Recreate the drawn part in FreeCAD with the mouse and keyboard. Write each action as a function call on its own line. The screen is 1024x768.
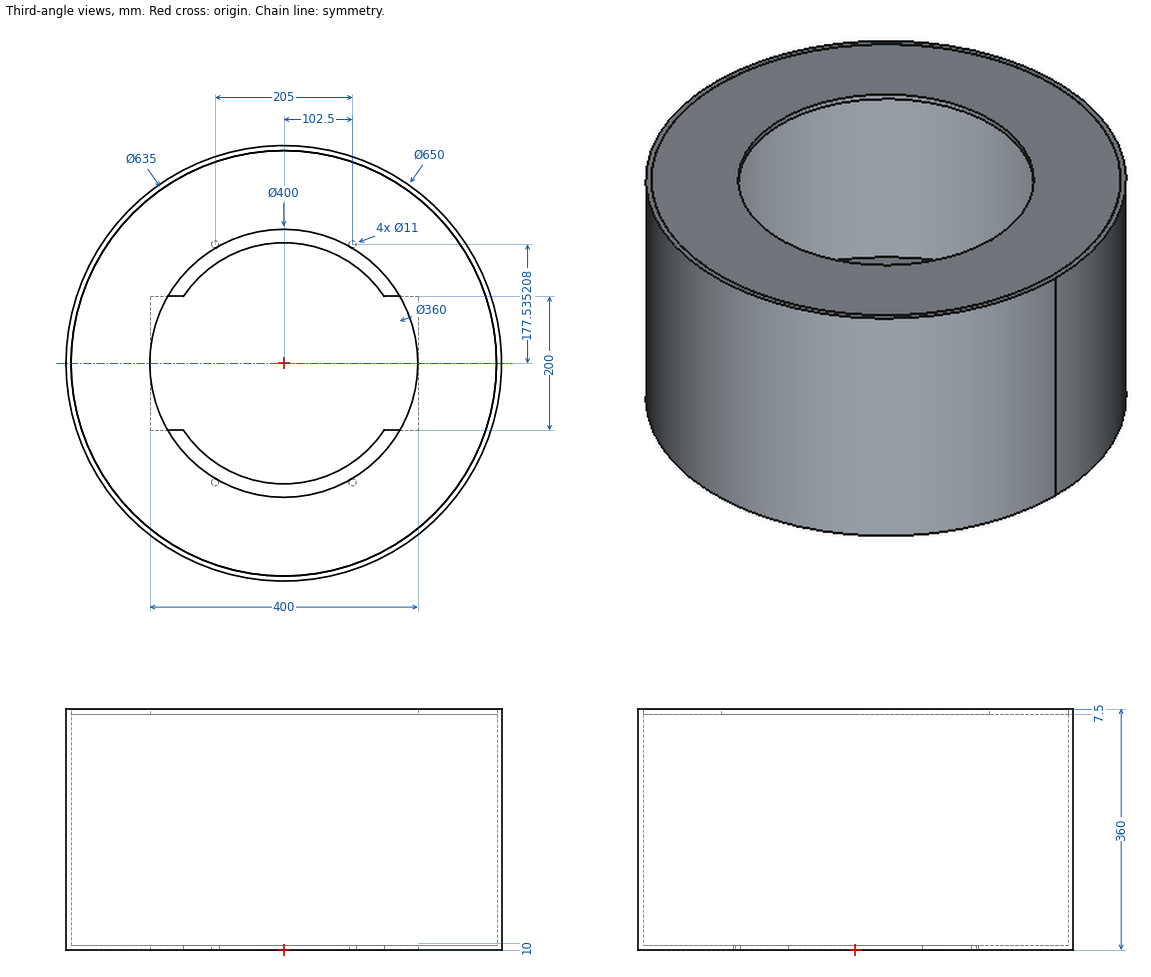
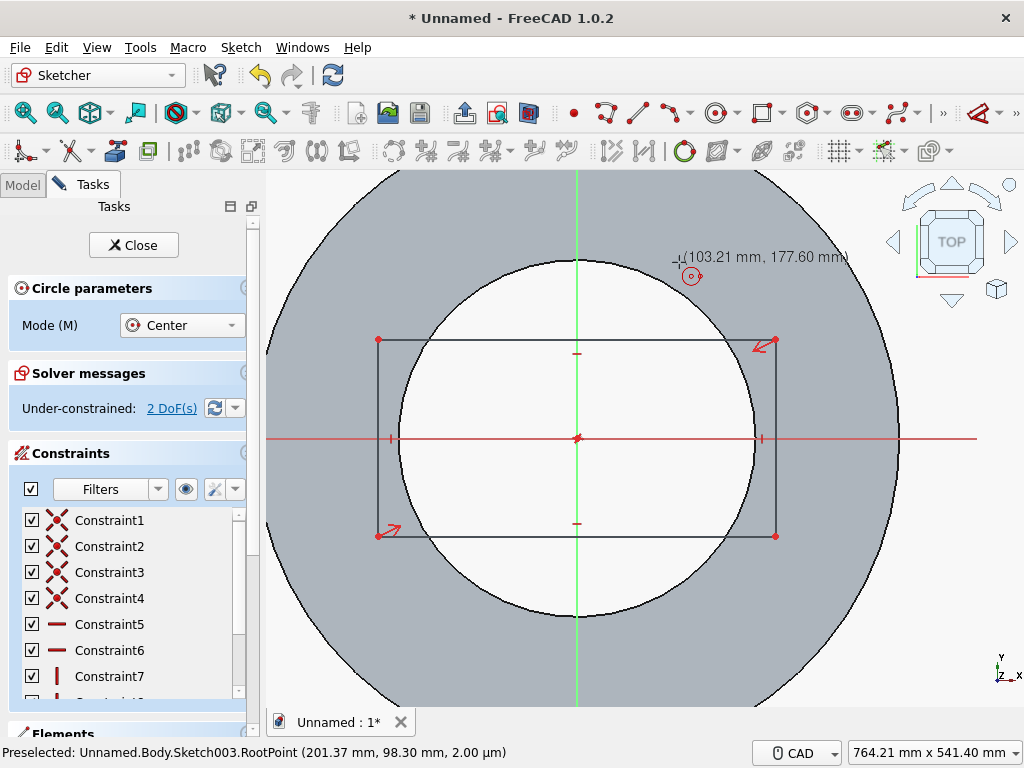
click(679, 262)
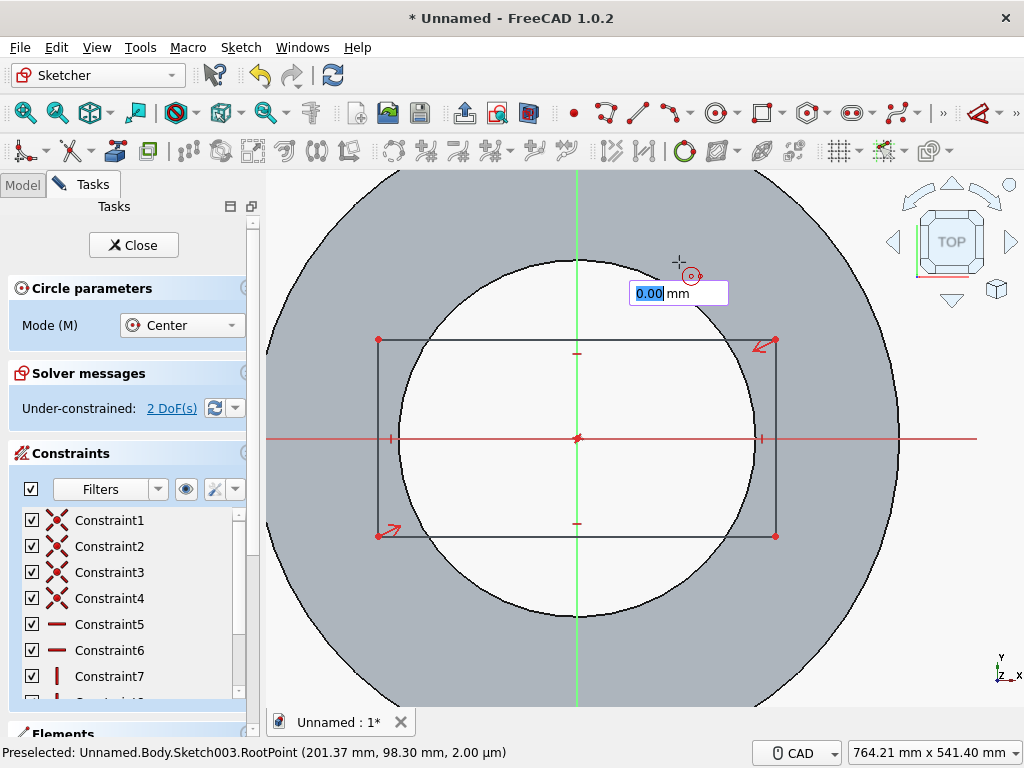
scroll(683, 259, up, 6)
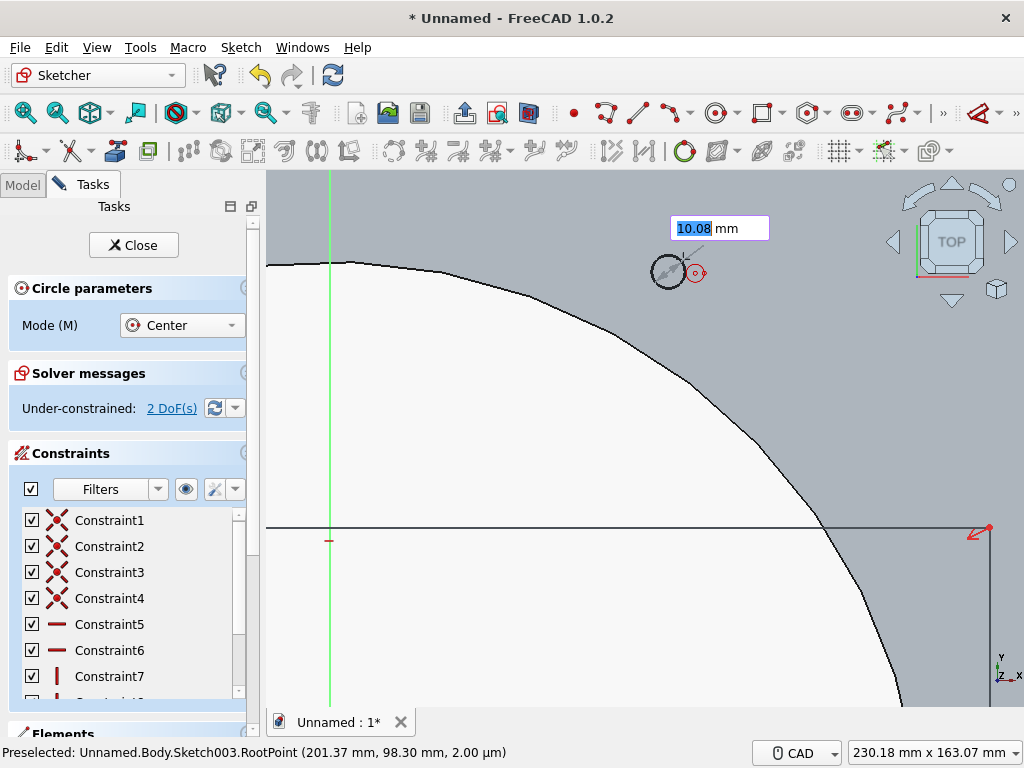
click(680, 257)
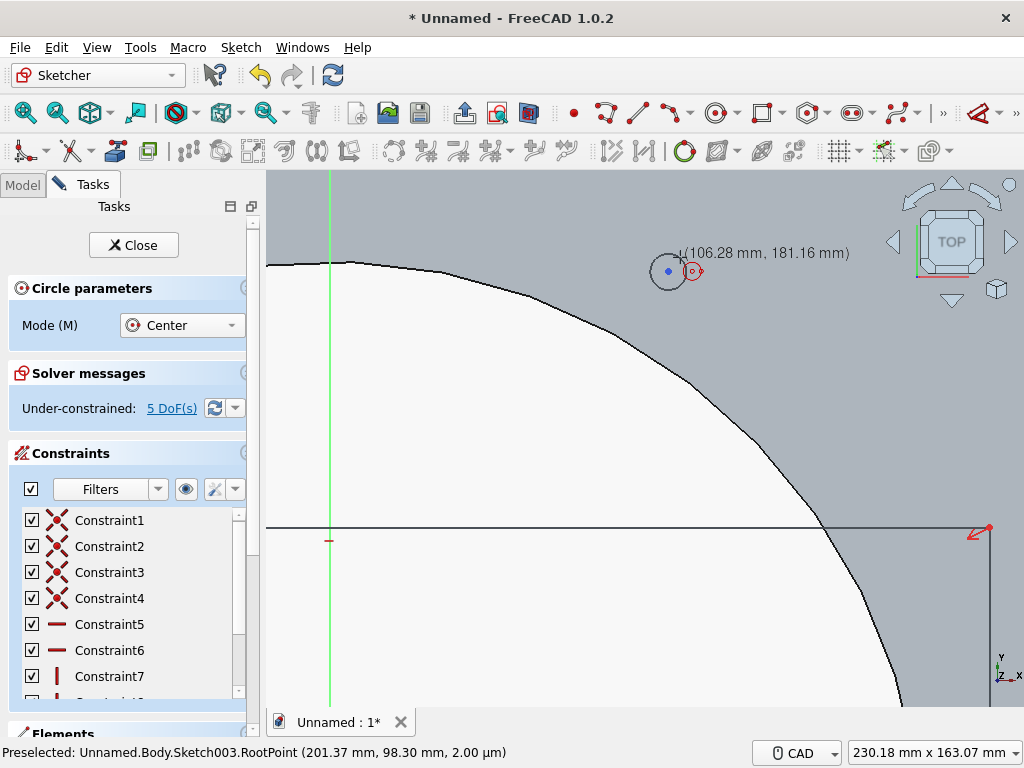
scroll(683, 259, down, 6)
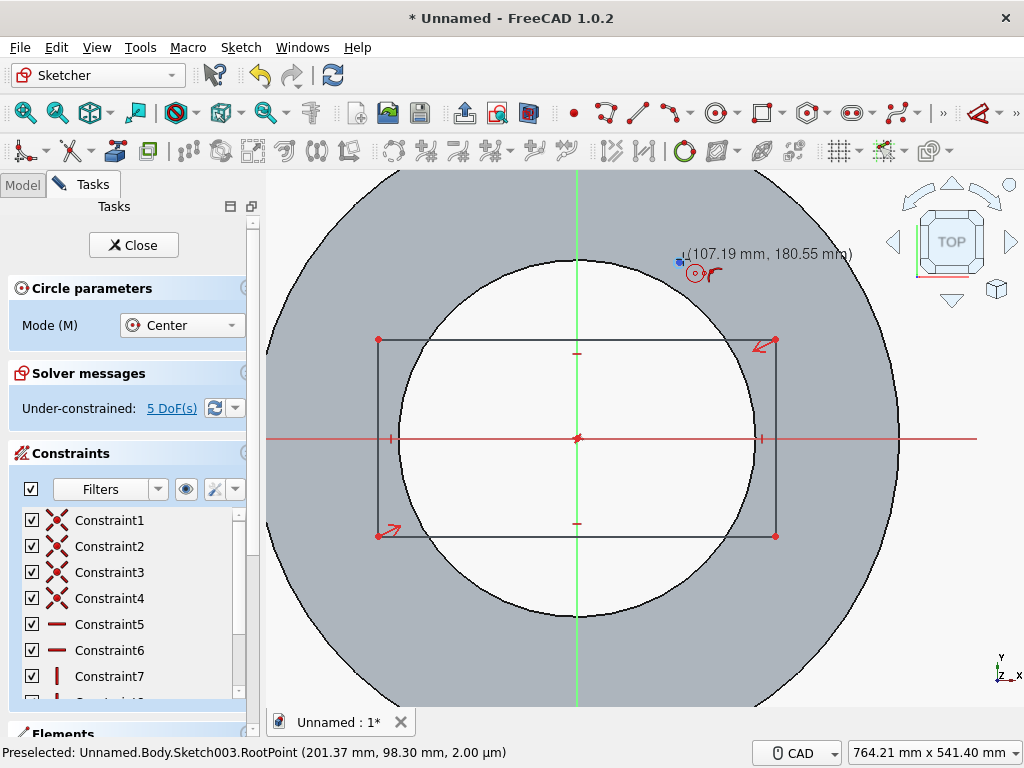
scroll(475, 262, up, 8)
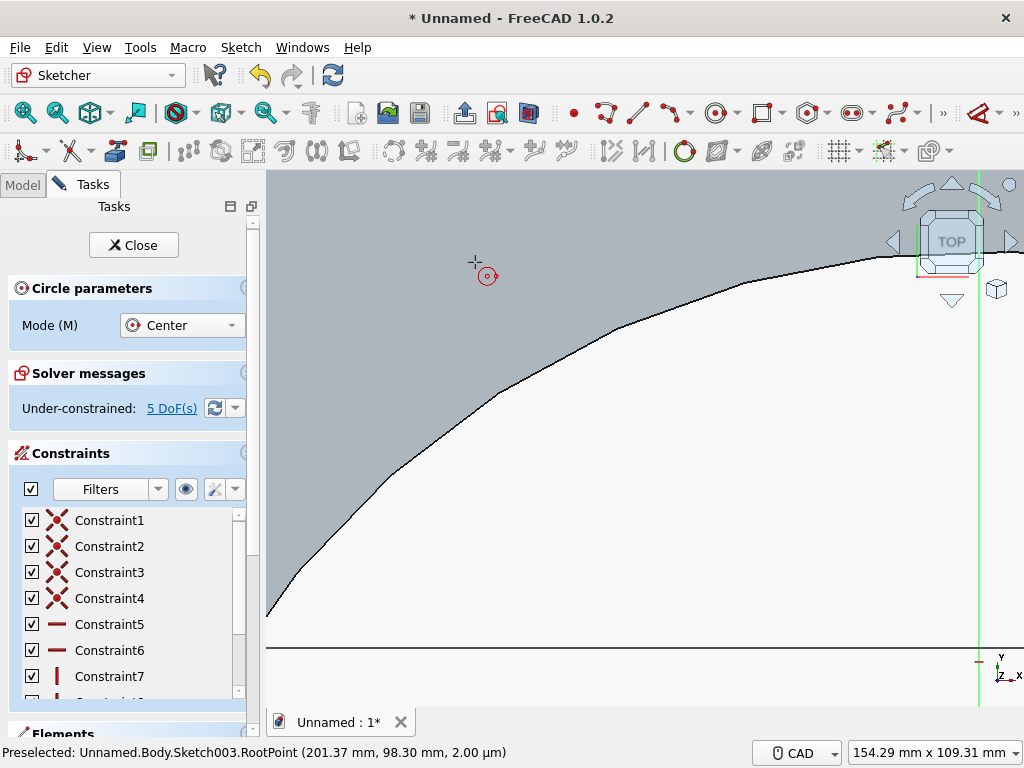
scroll(475, 262, down, 8)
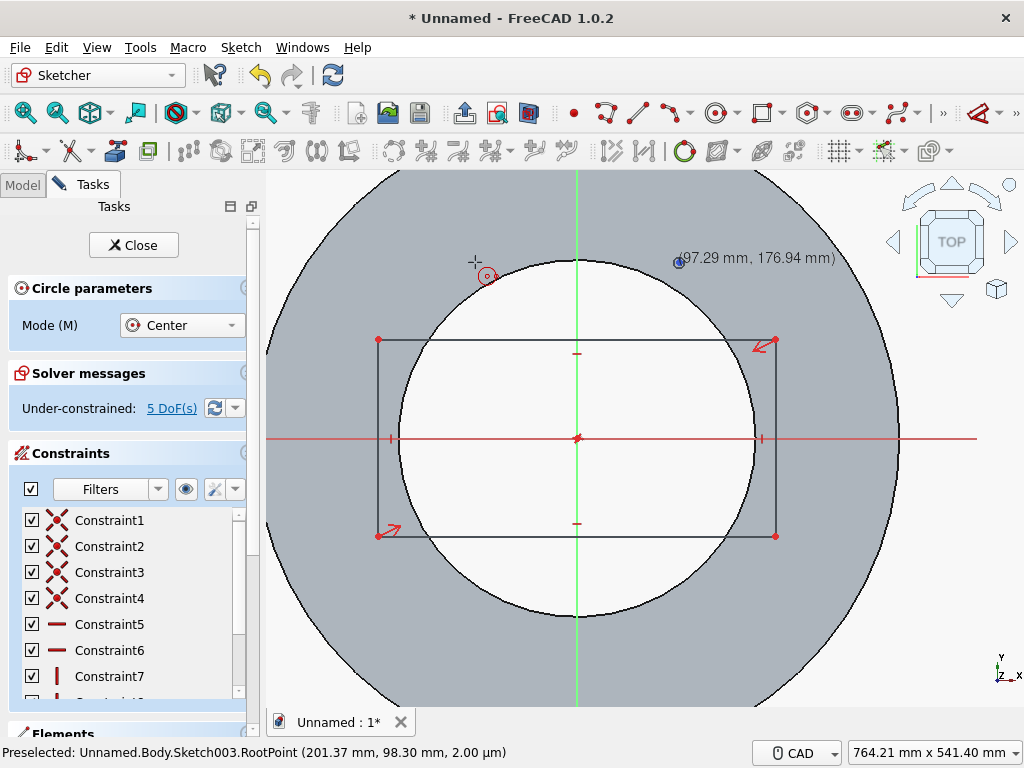
click(475, 262)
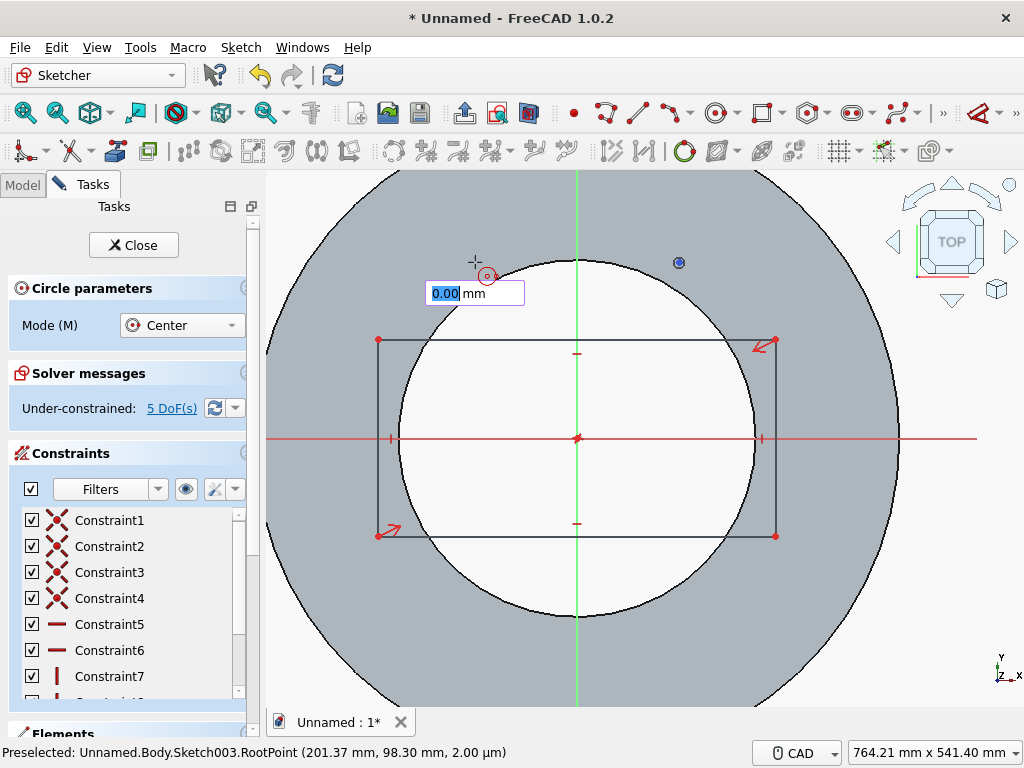
scroll(479, 259, up, 6)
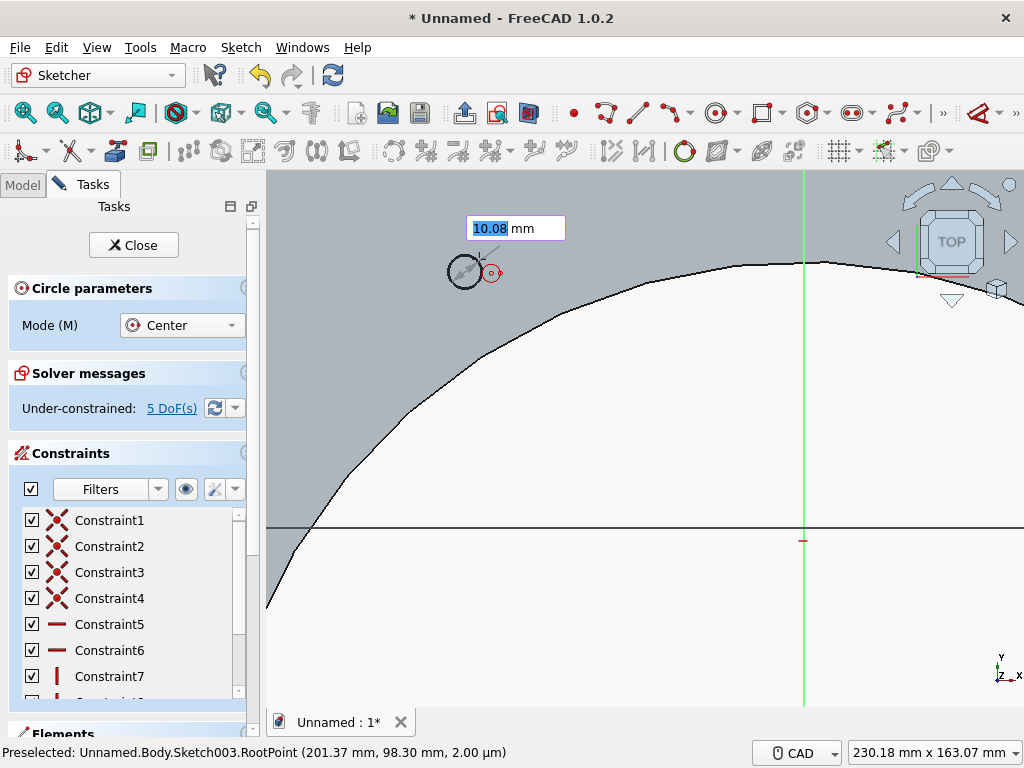
click(479, 257)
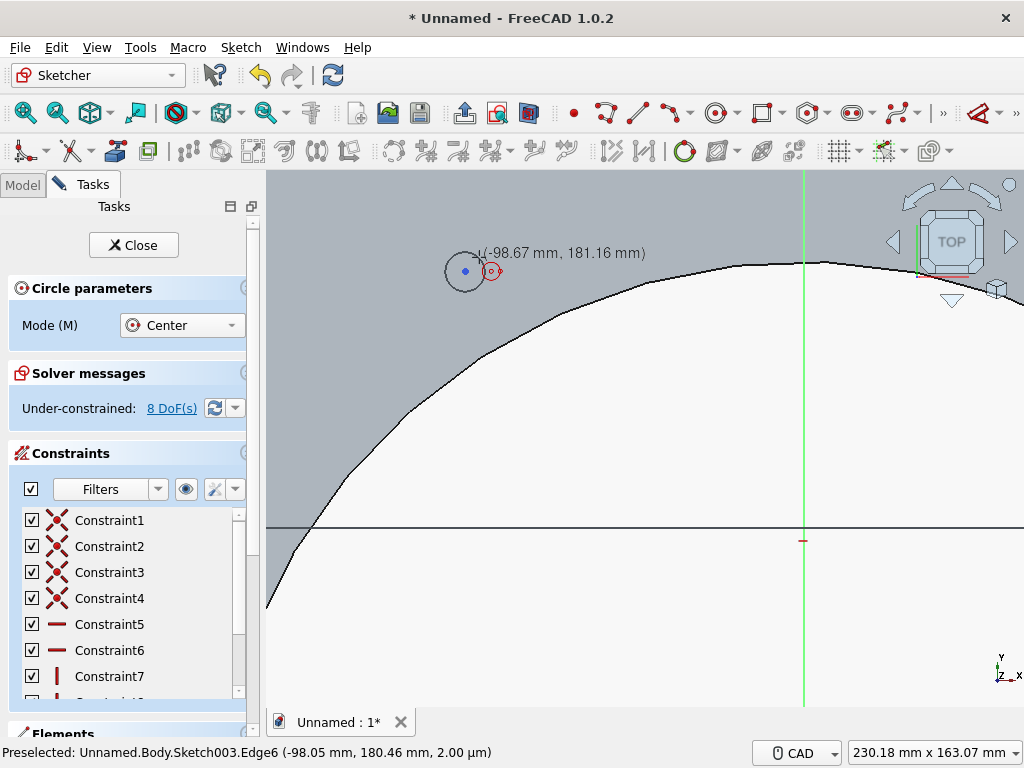
scroll(478, 259, down, 6)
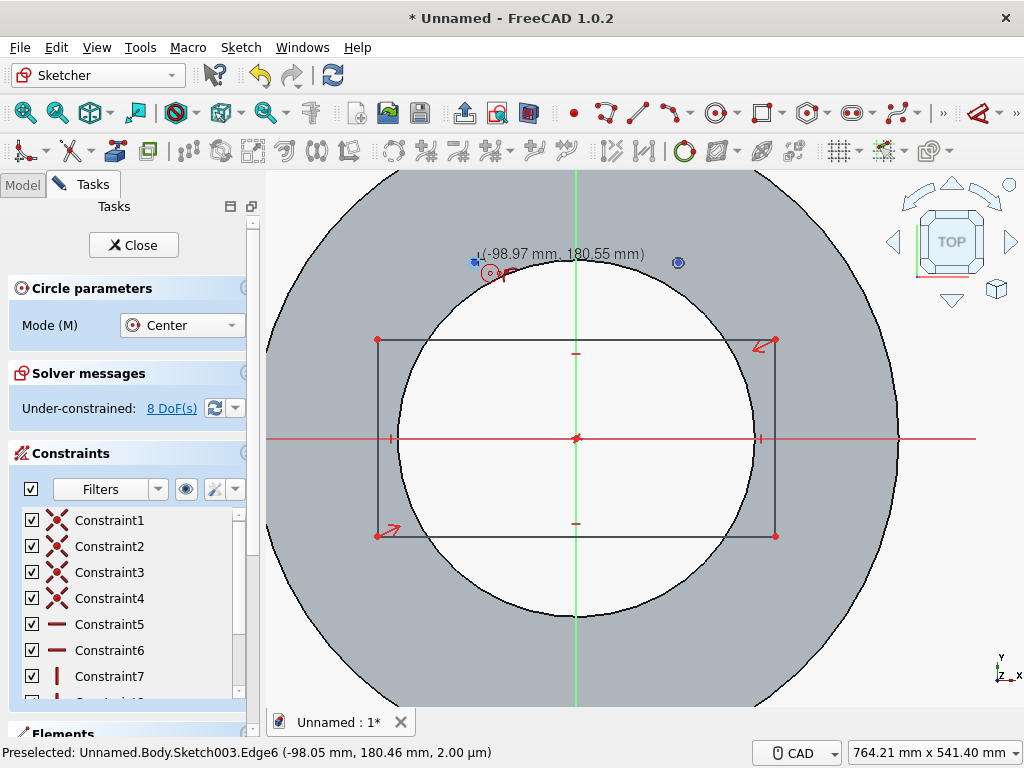
scroll(475, 615, up, 8)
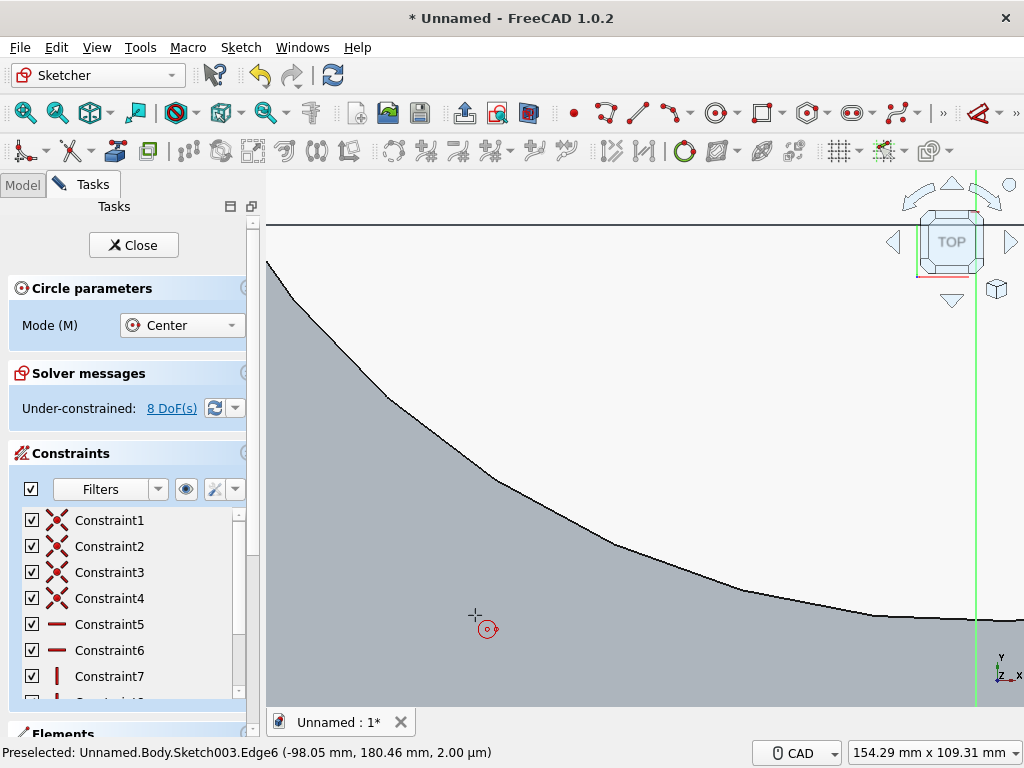
scroll(475, 616, down, 8)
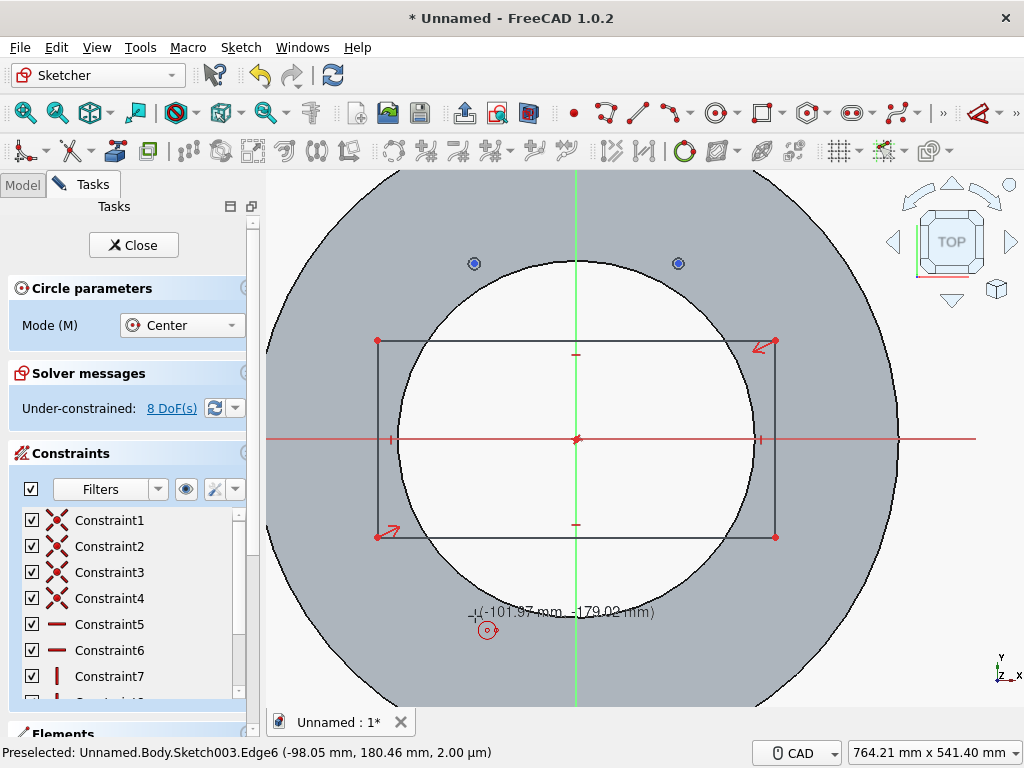
click(475, 615)